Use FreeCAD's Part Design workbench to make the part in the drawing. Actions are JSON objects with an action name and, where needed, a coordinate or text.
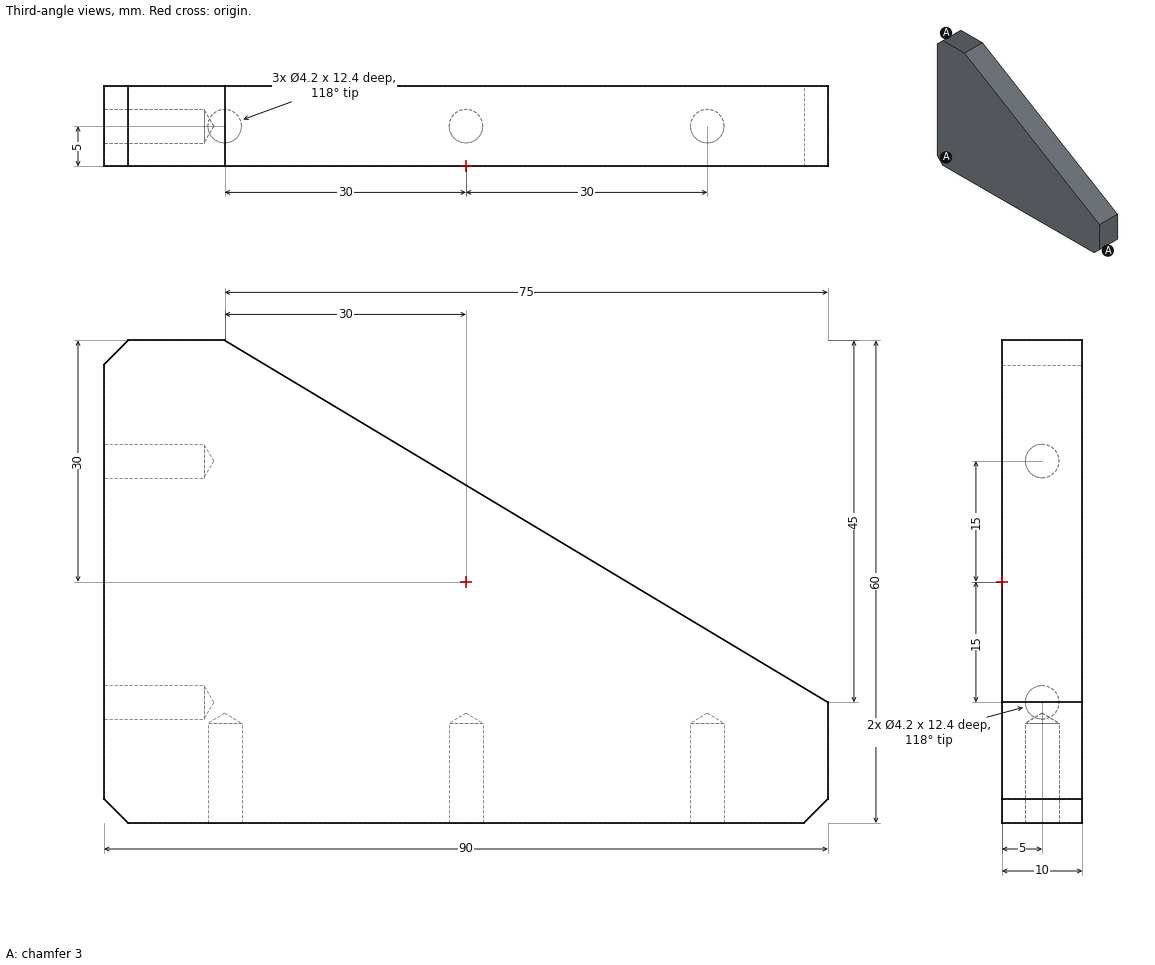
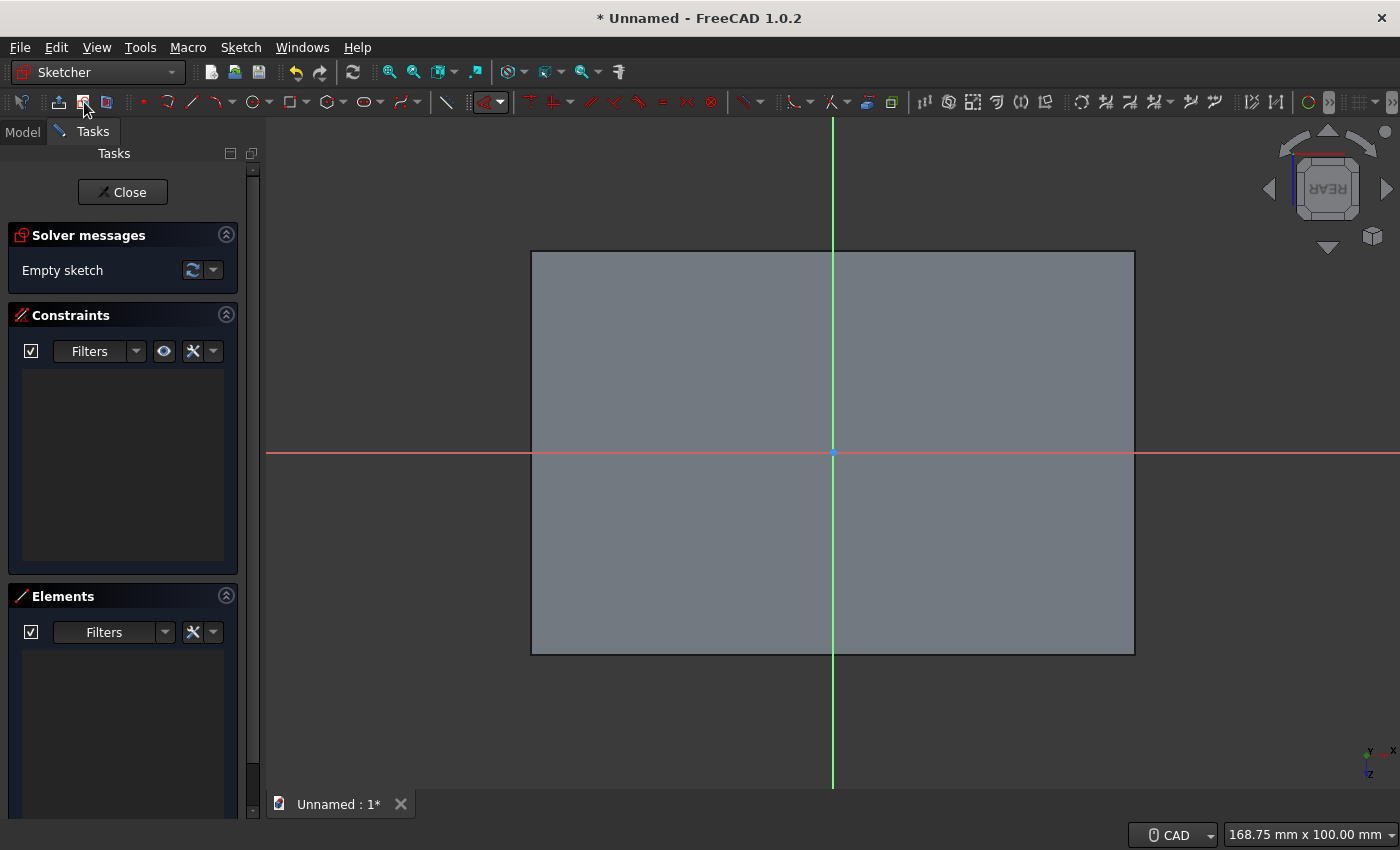
{"action": "left_click", "coordinate": [631, 655]}
{"action": "left_click", "coordinate": [1135, 655]}
{"action": "left_click", "coordinate": [1135, 352]}
{"action": "left_click", "coordinate": [631, 656]}
{"action": "key", "text": "Escape"}
{"action": "key", "text": "Escape"}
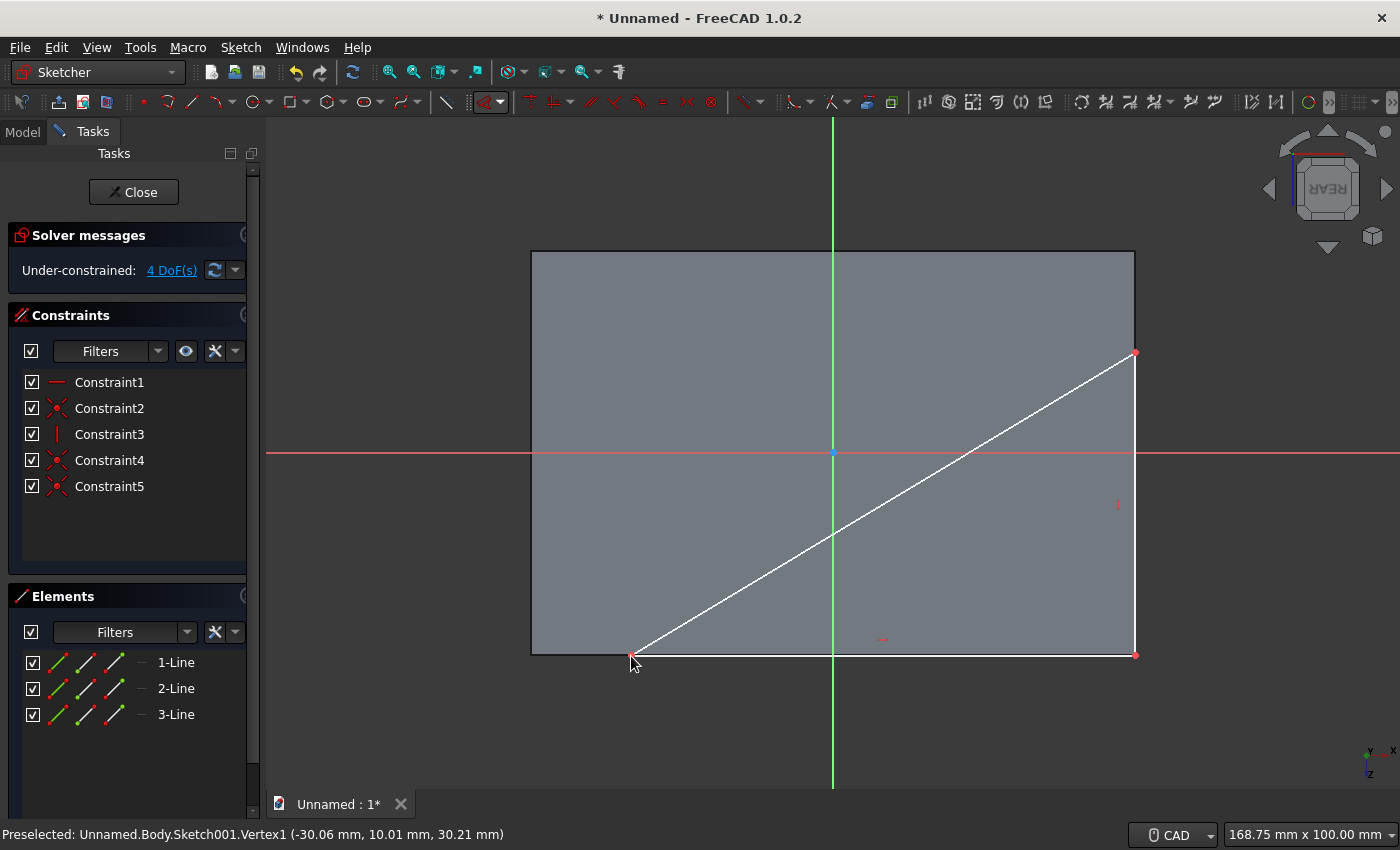
{"action": "key", "text": "d"}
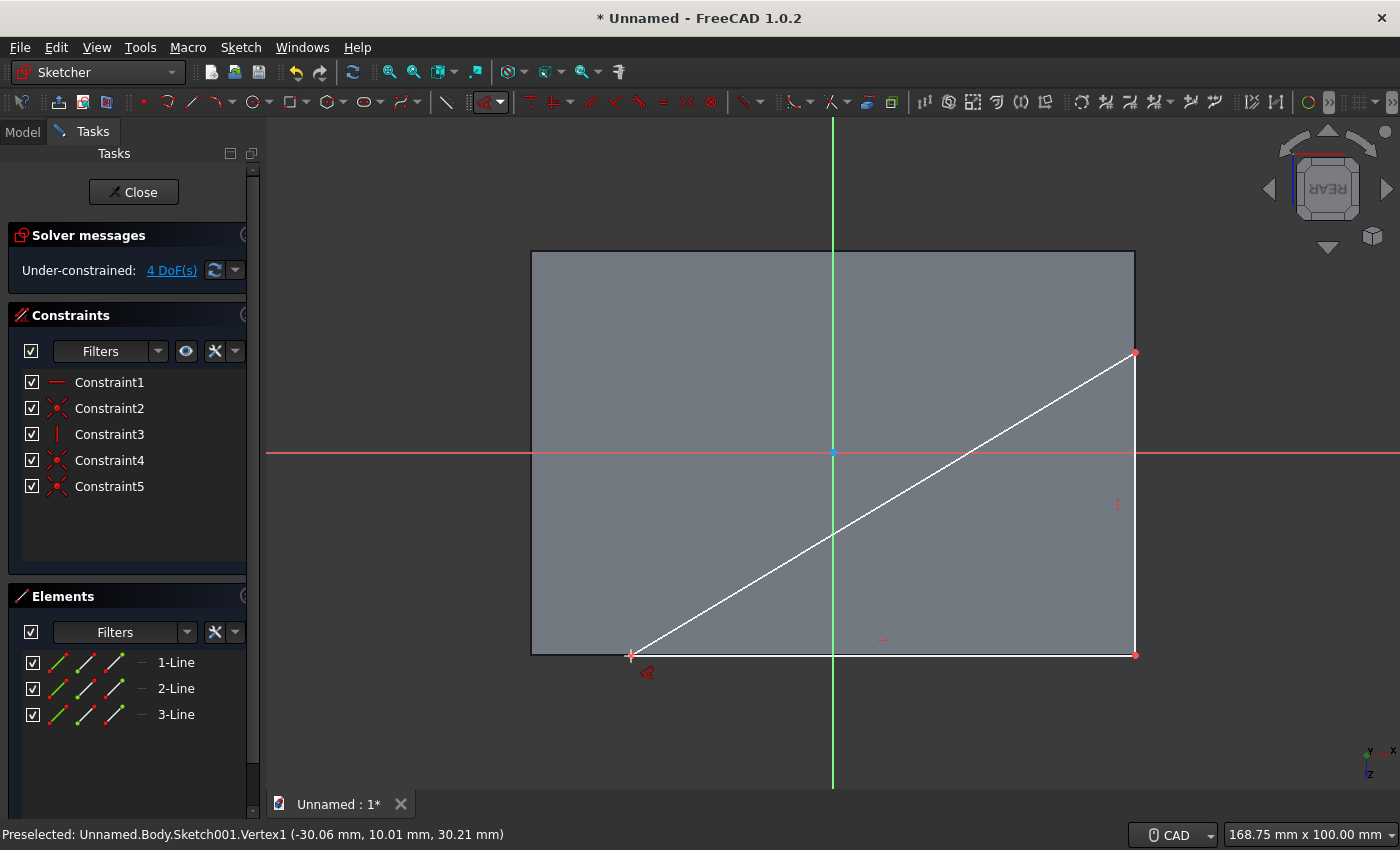
{"action": "left_click", "coordinate": [782, 656]}
{"action": "left_click", "coordinate": [883, 690]}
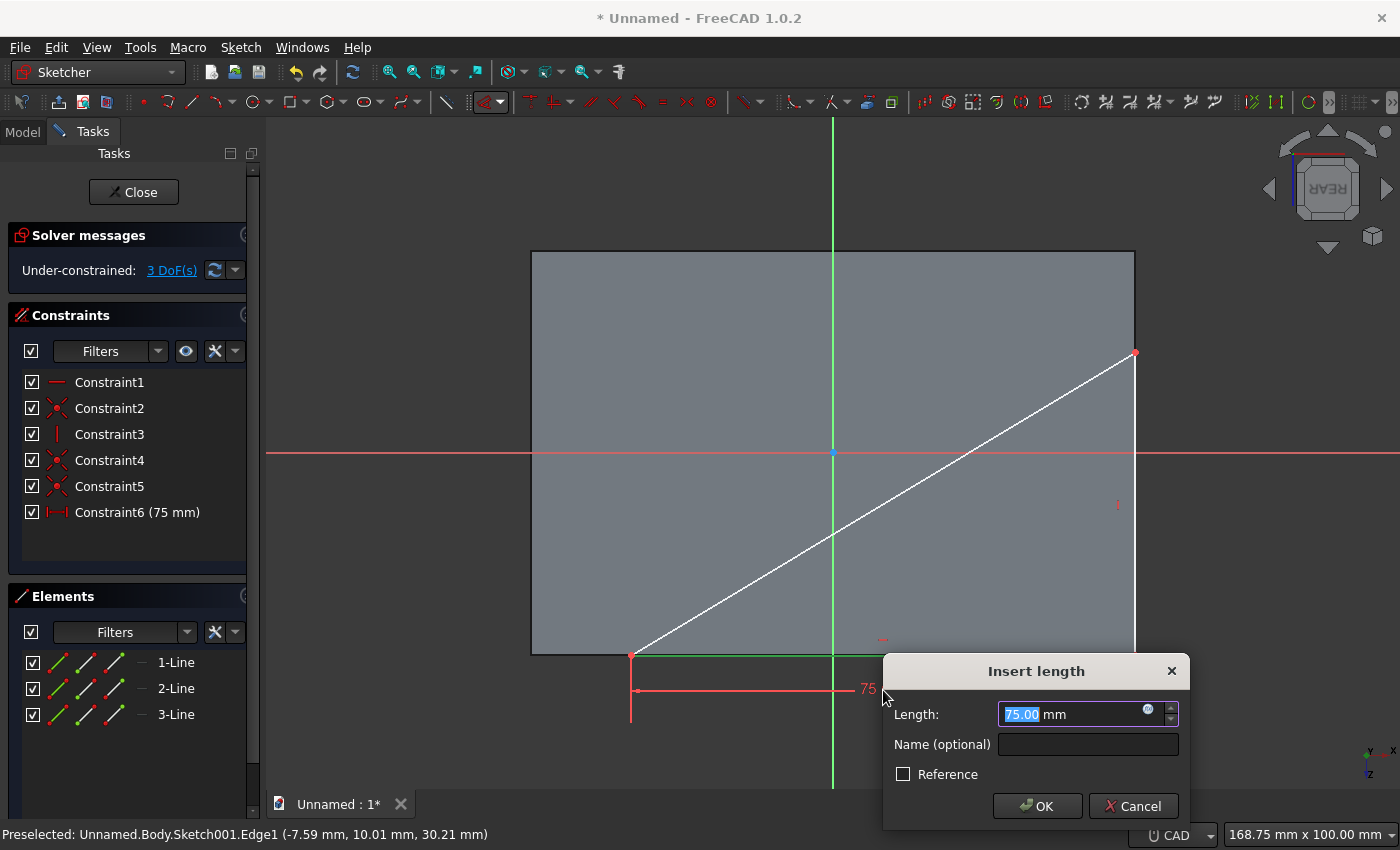
{"action": "type", "text": "75"}
{"action": "key", "text": "Return"}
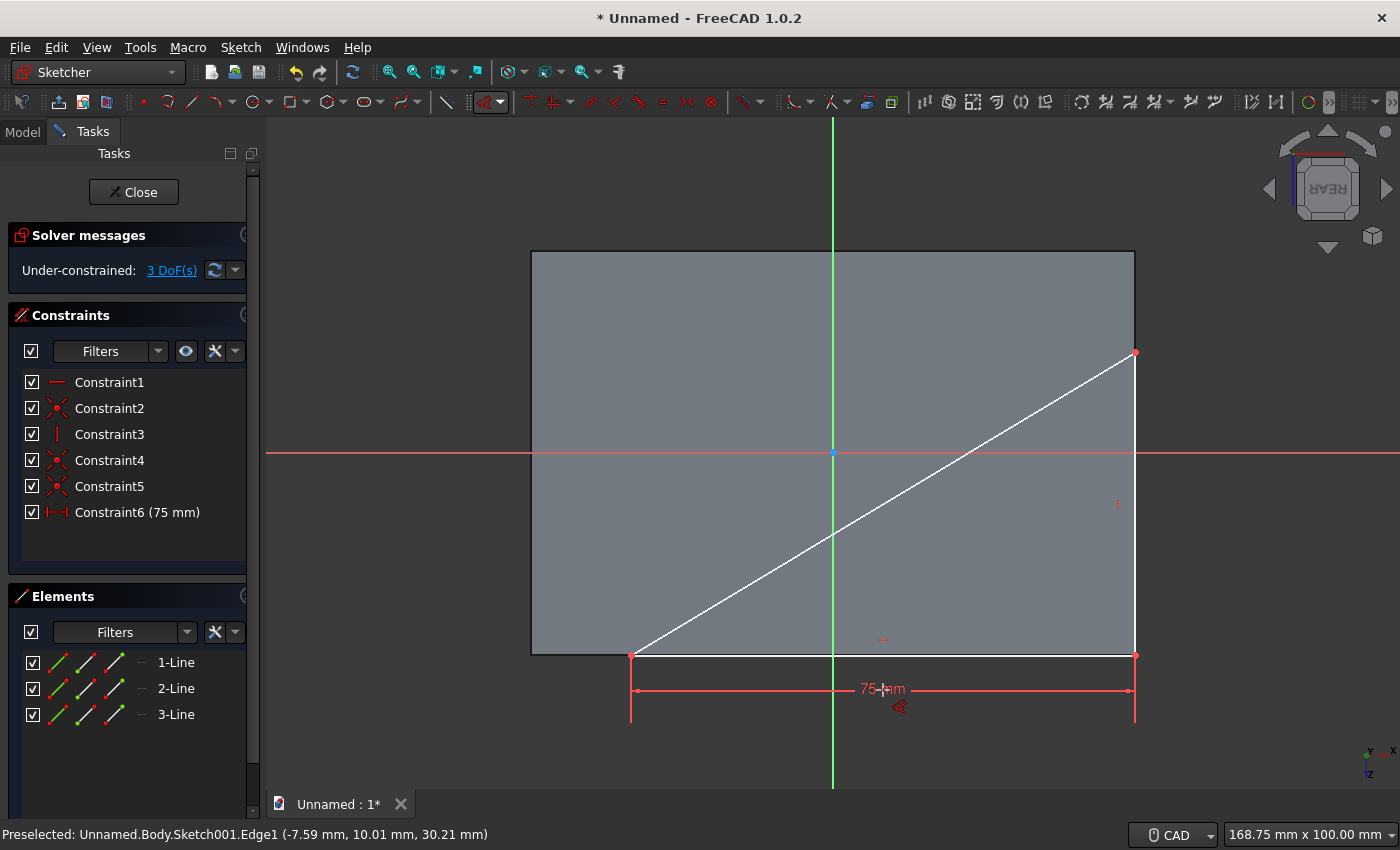
{"action": "left_click", "coordinate": [1135, 565]}
{"action": "left_click", "coordinate": [1169, 504]}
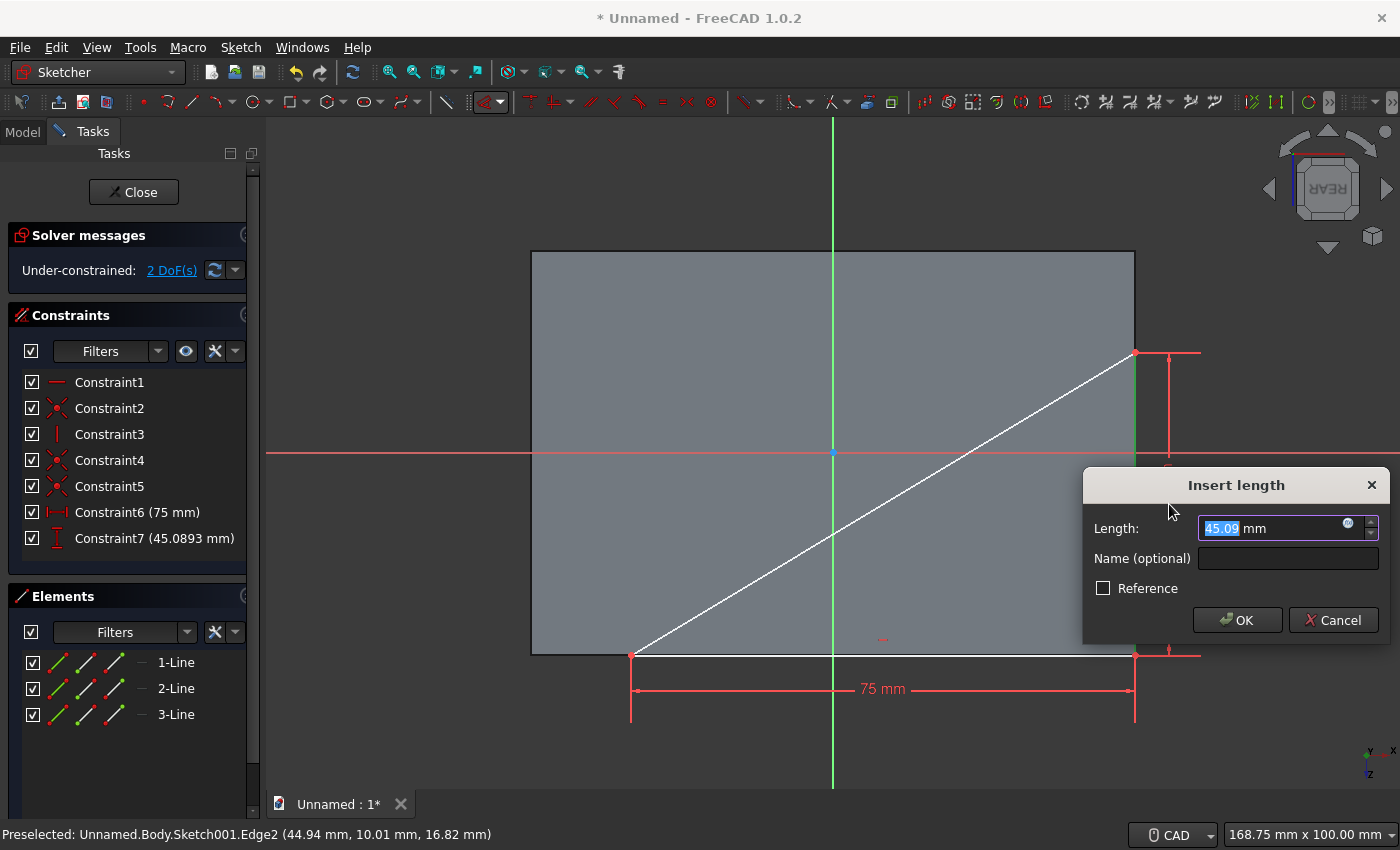
{"action": "type", "text": "45"}
{"action": "key", "text": "Return"}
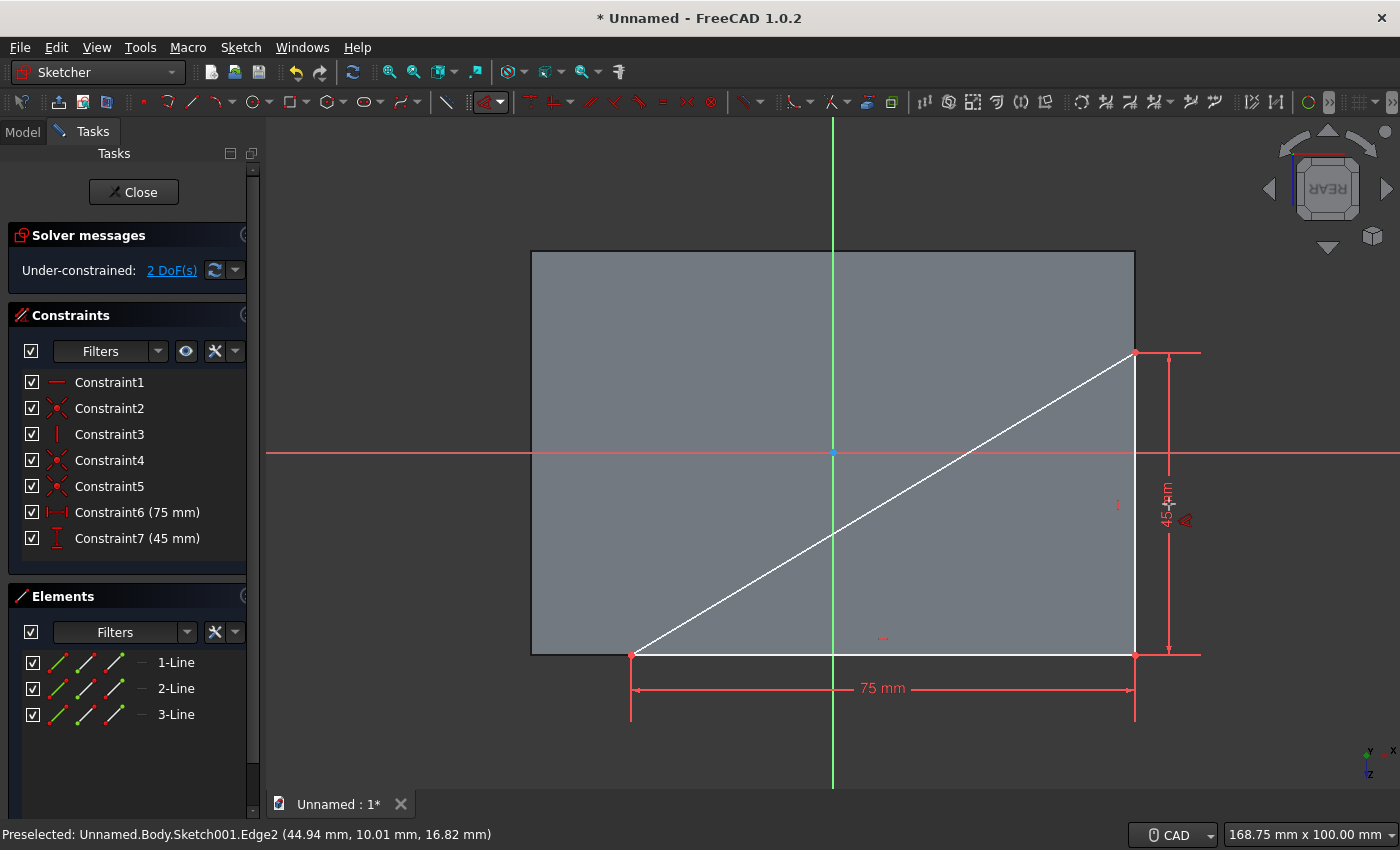
{"action": "left_click", "coordinate": [631, 655]}
{"action": "left_click", "coordinate": [732, 689]}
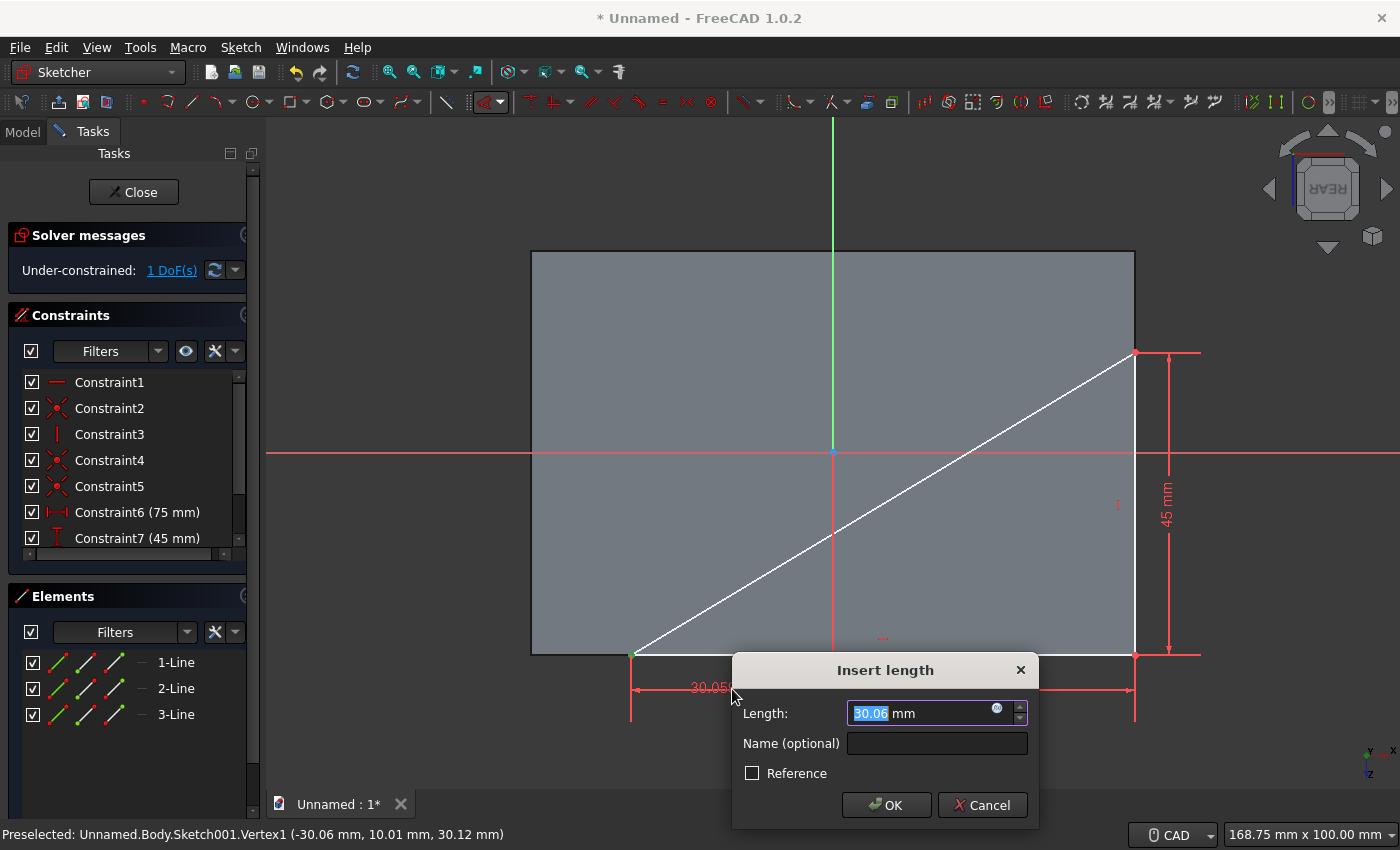
{"action": "type", "text": "30"}
{"action": "key", "text": "Return"}